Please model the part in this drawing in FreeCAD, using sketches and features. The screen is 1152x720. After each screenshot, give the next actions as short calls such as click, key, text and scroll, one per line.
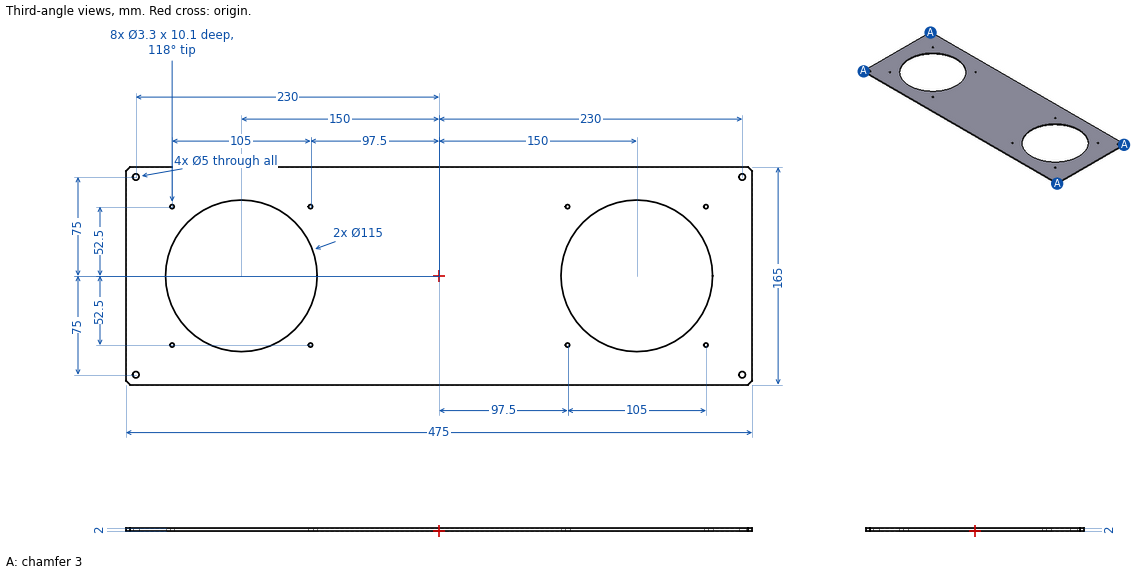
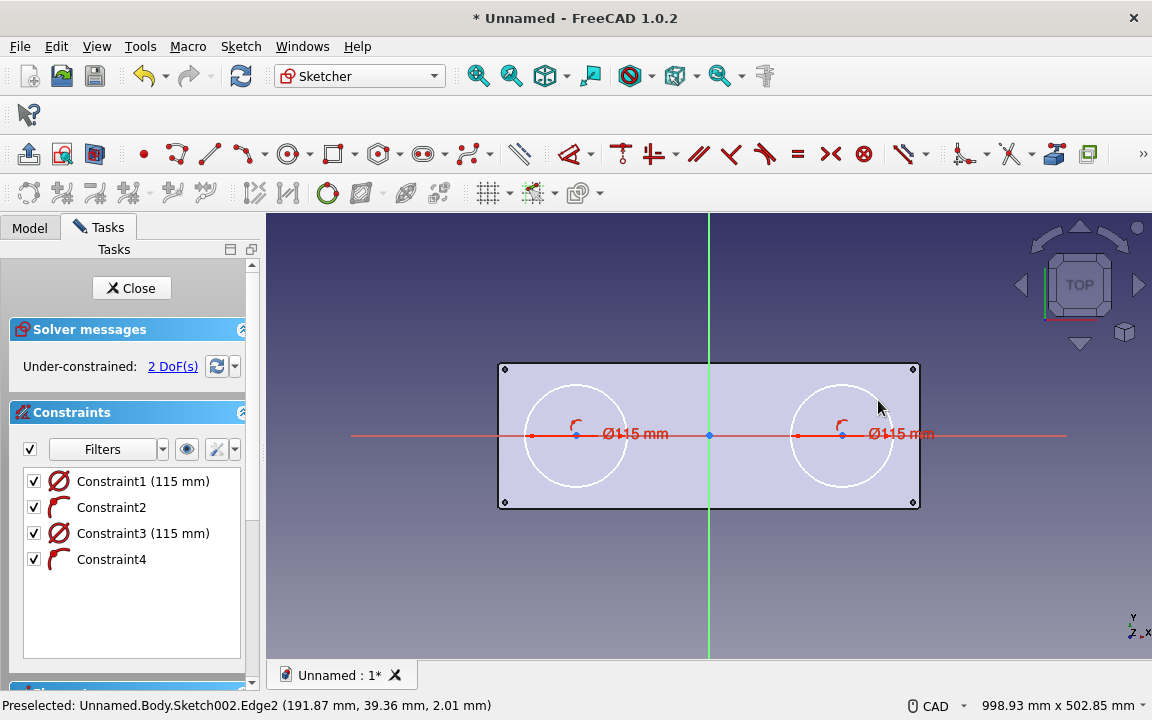
key(d)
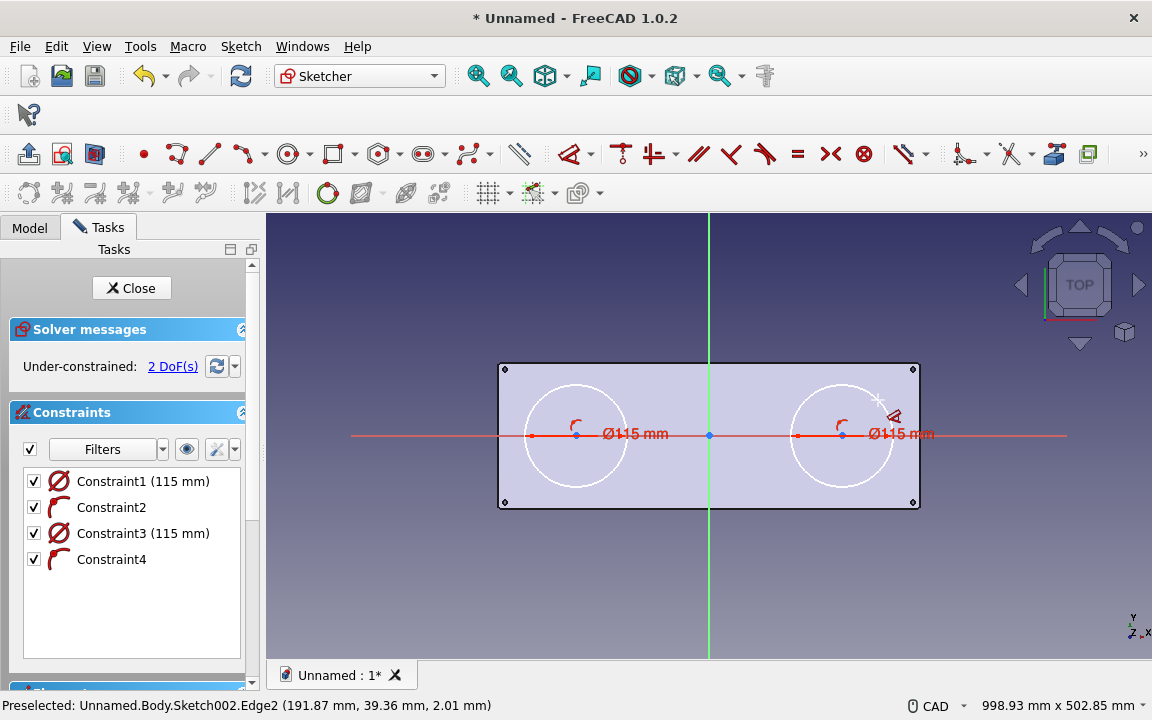
click(576, 436)
click(643, 470)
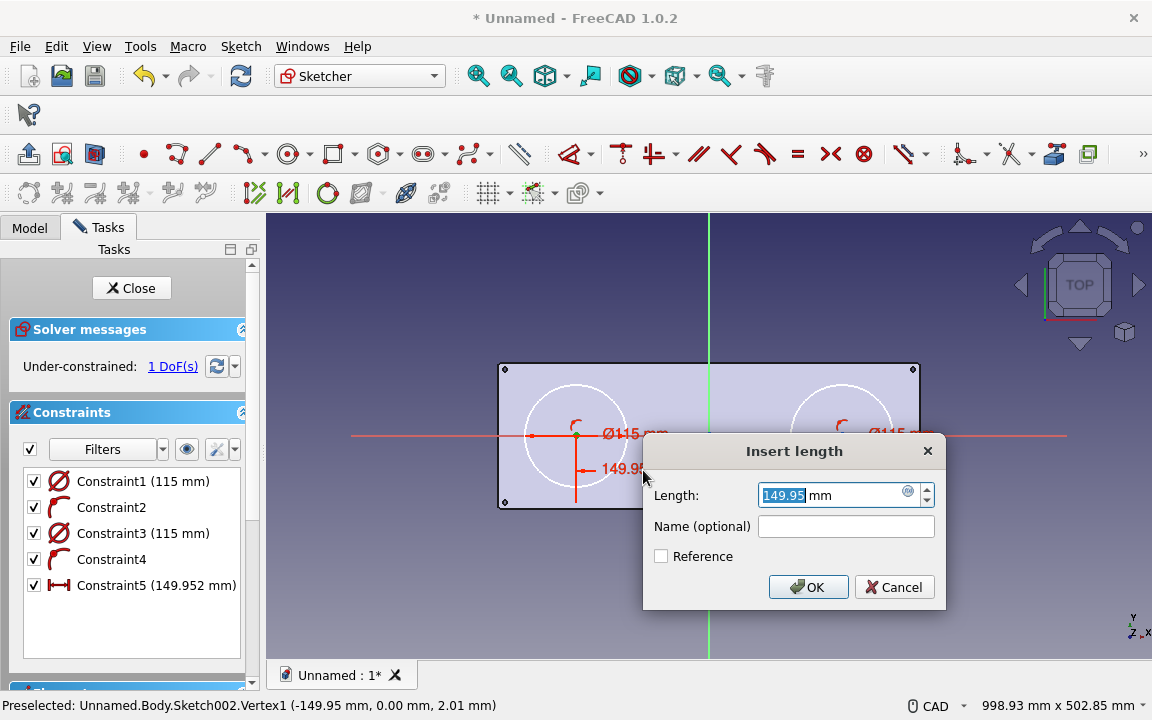
text(150)
key(Return)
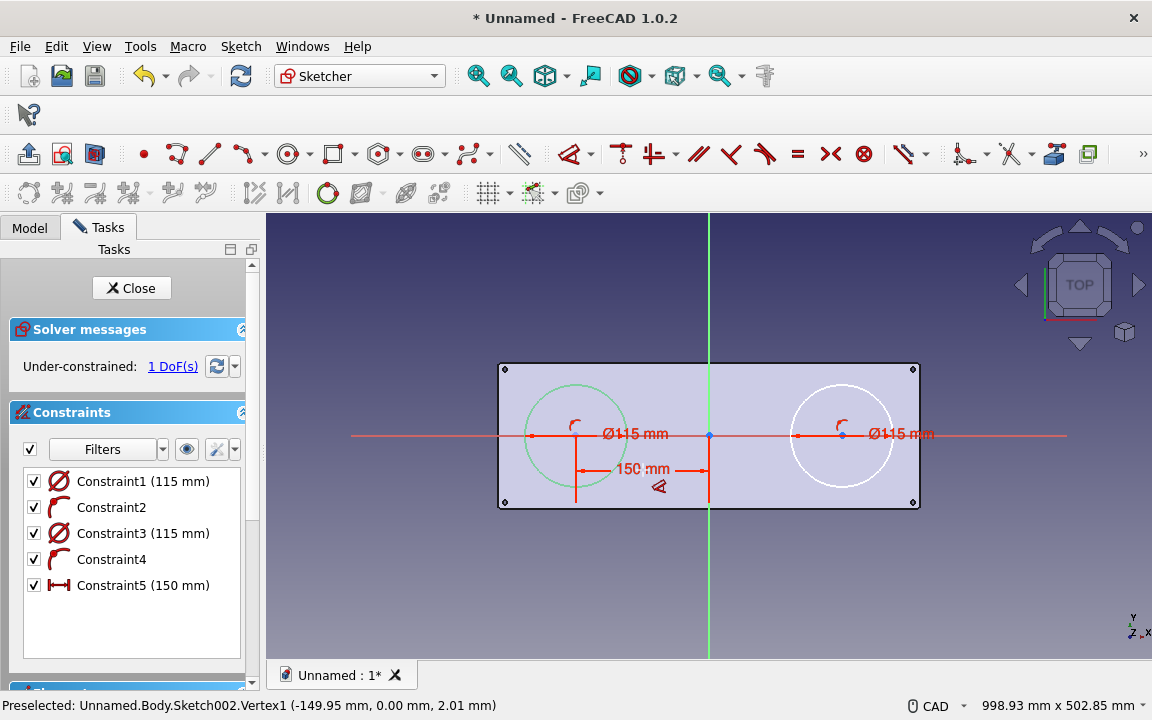
click(842, 436)
click(775, 470)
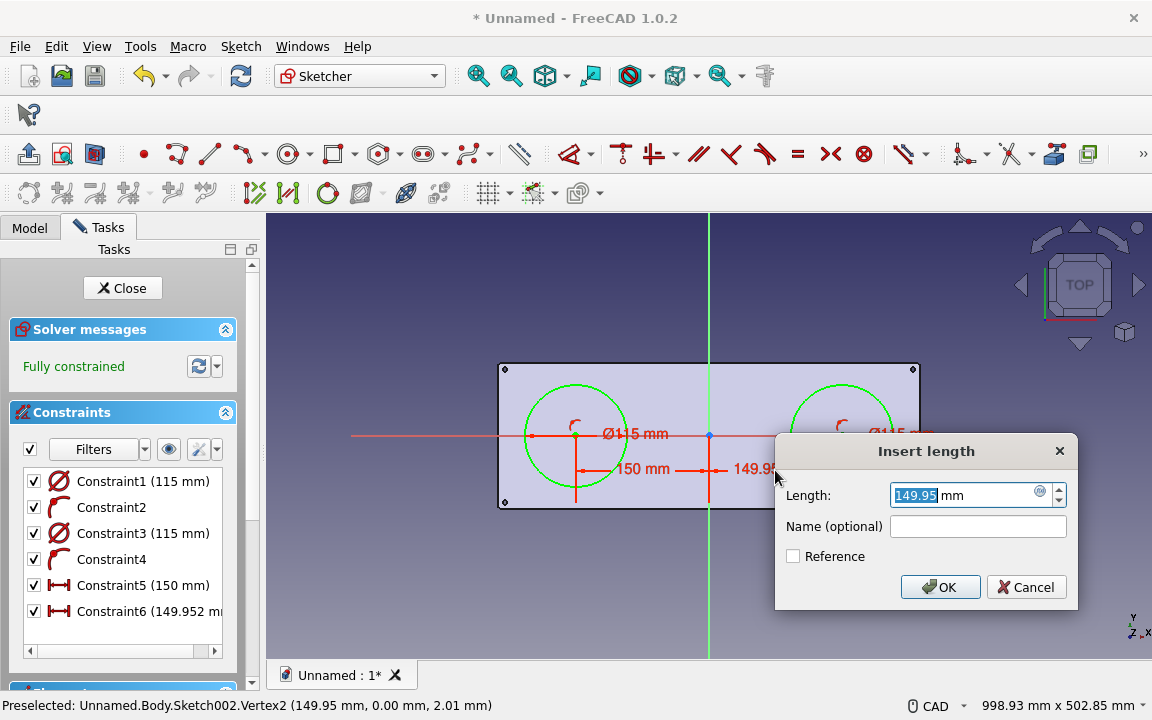
text(150)
key(Return)
key(Escape)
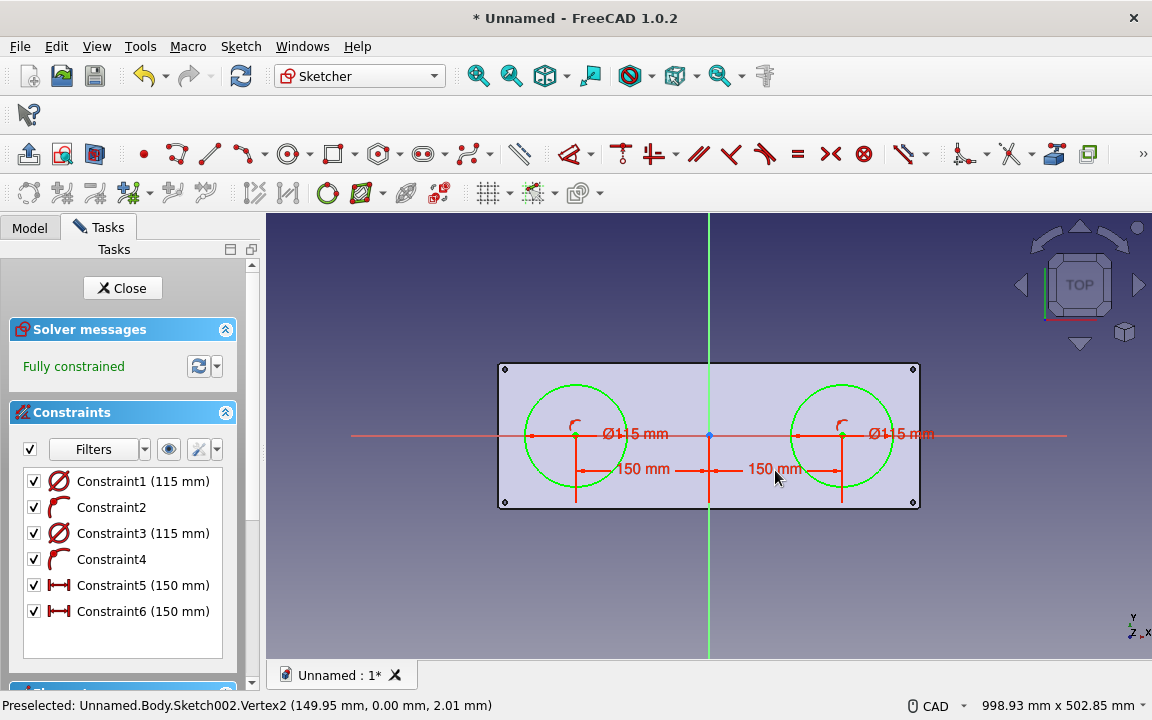
click(123, 288)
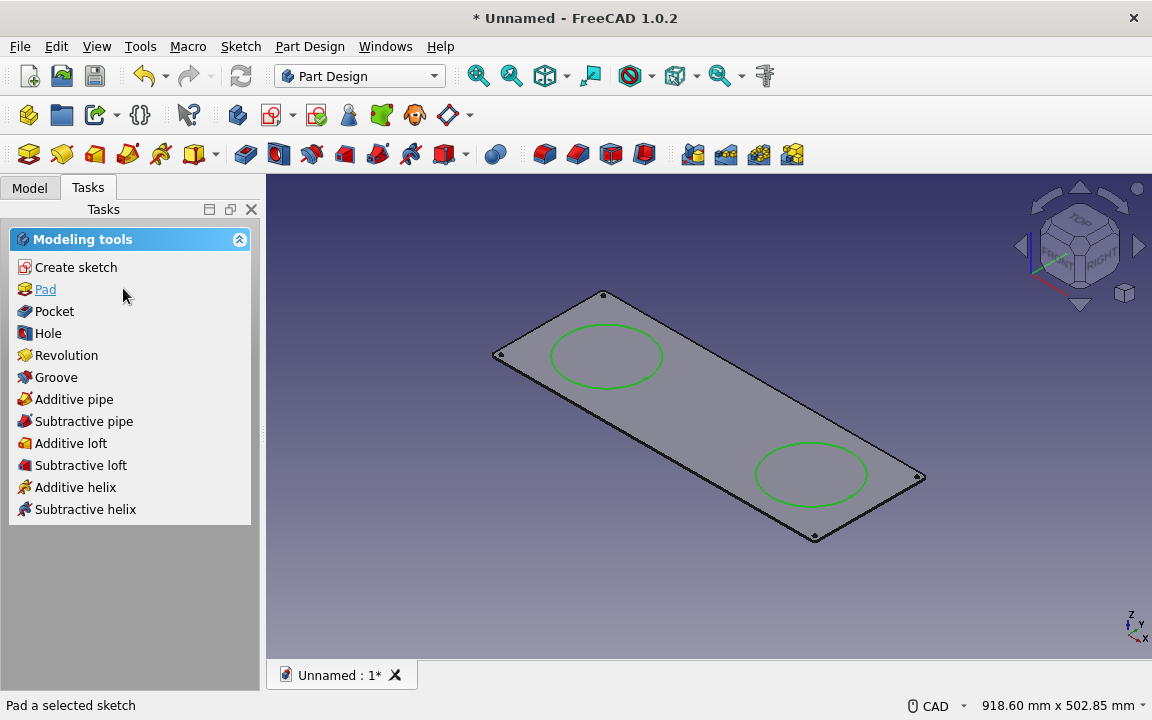
click(246, 154)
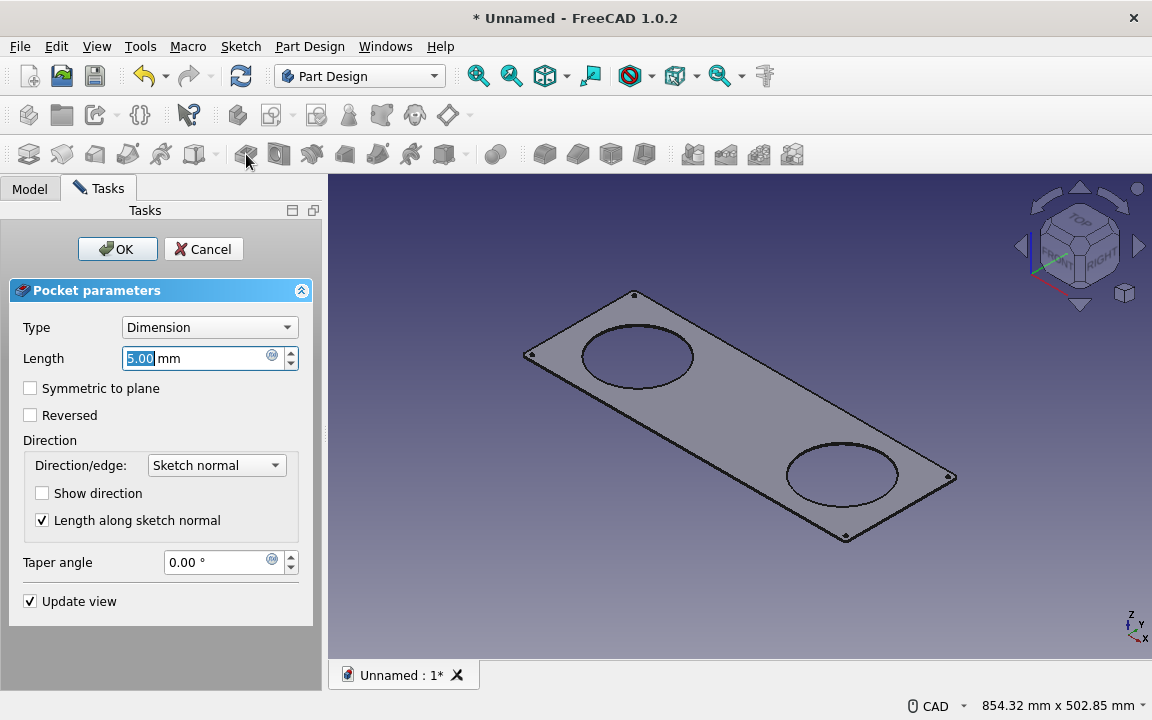
text(2)
key(Tab)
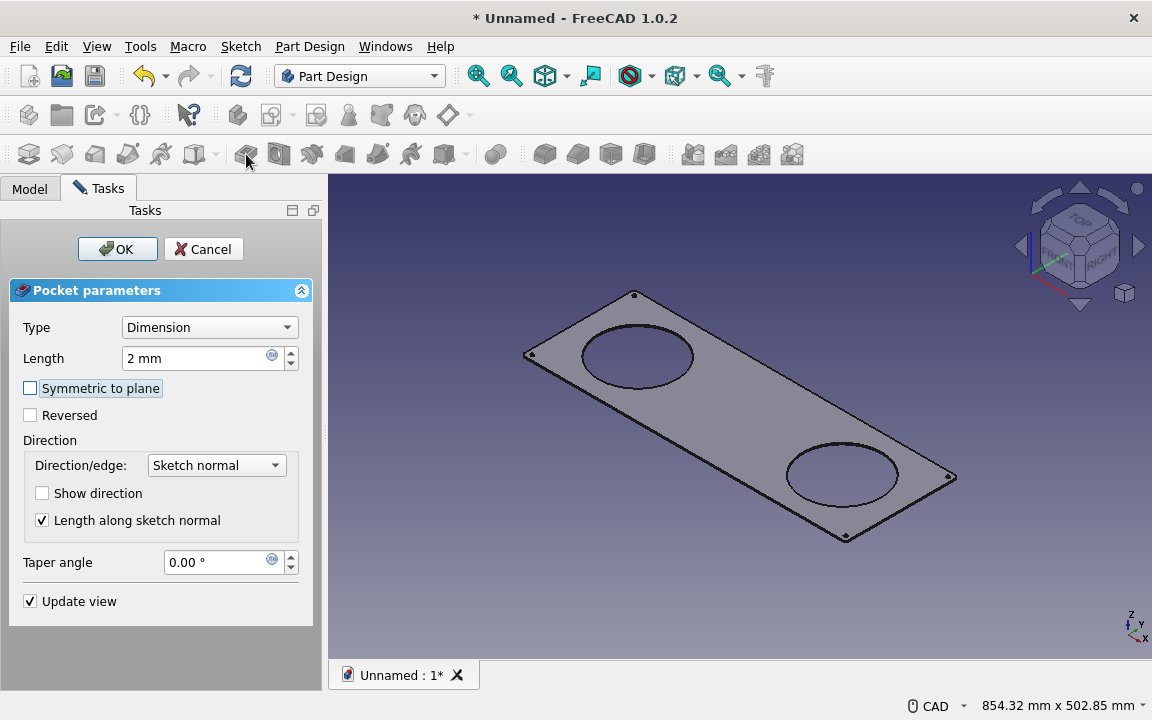
click(118, 249)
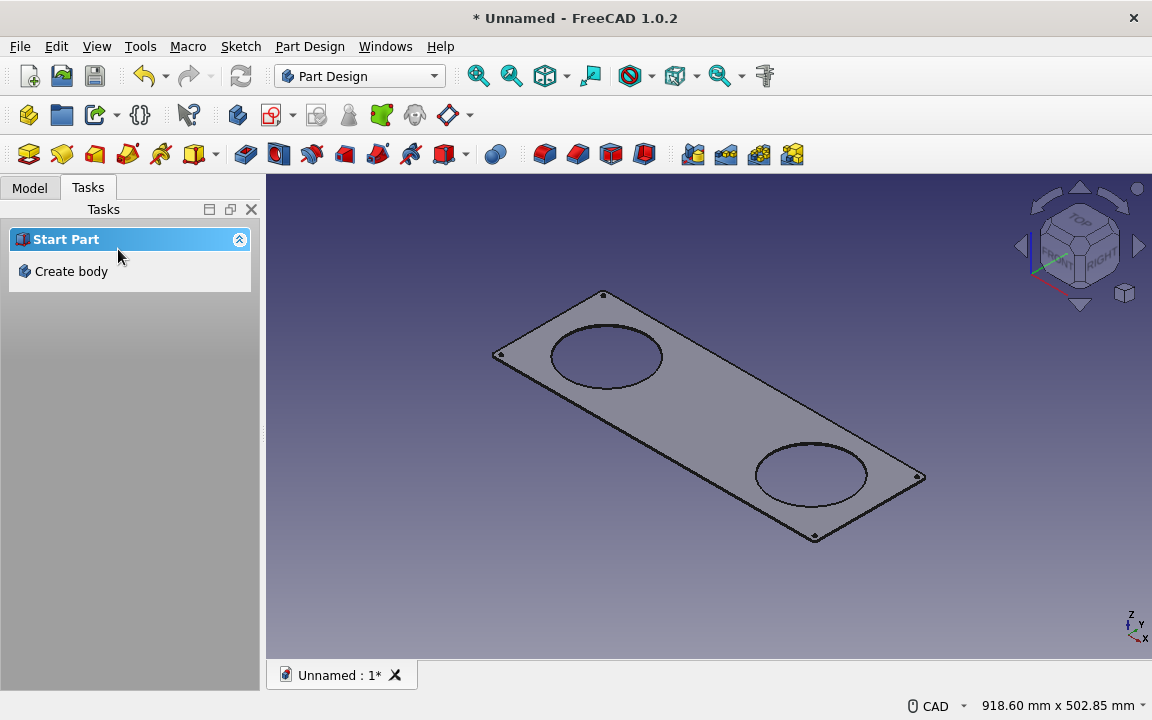
click(709, 415)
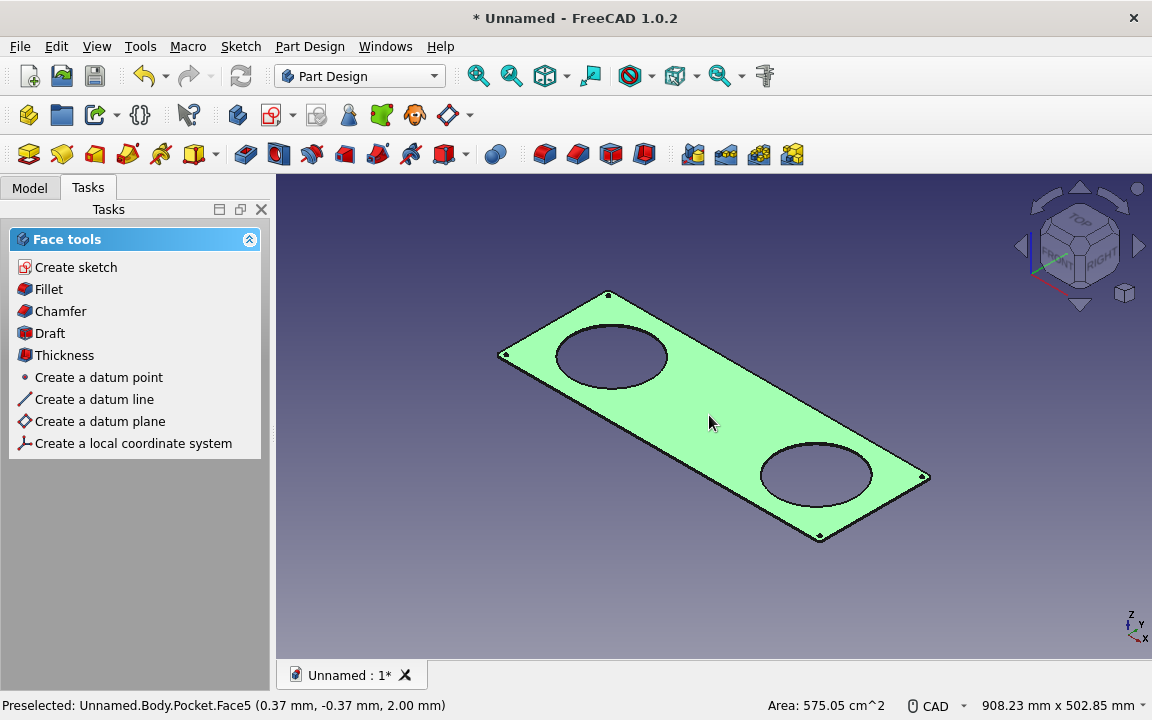
click(270, 116)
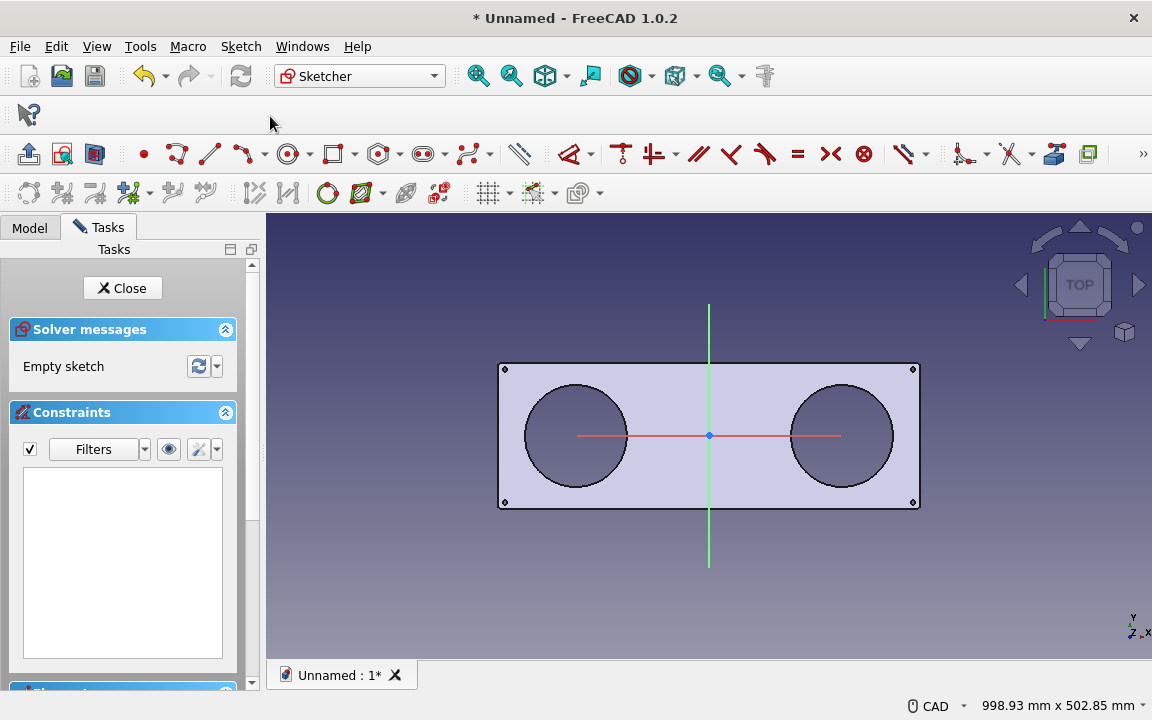
scroll(848, 436, up, 2)